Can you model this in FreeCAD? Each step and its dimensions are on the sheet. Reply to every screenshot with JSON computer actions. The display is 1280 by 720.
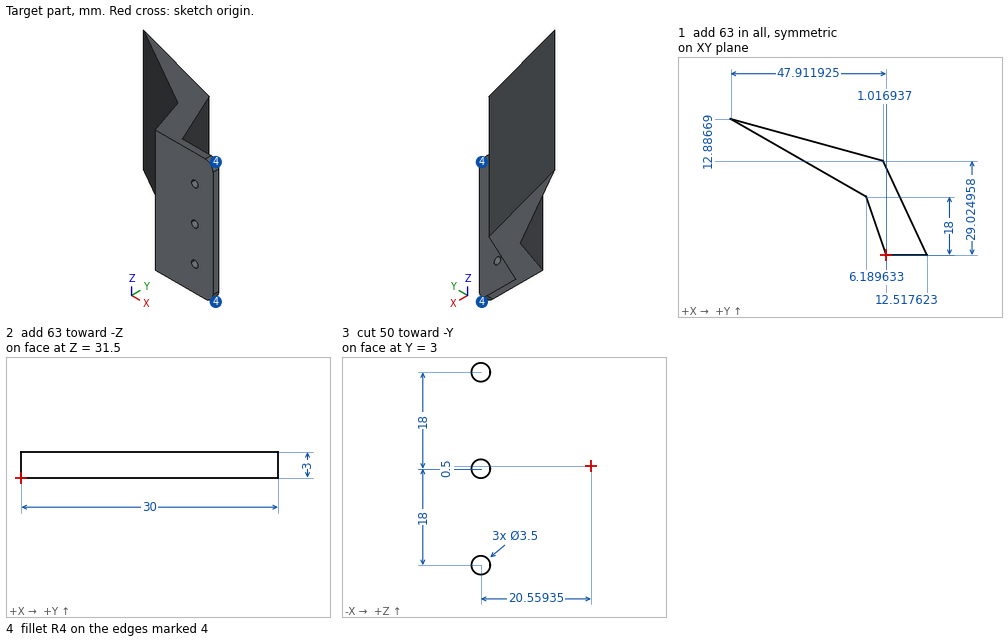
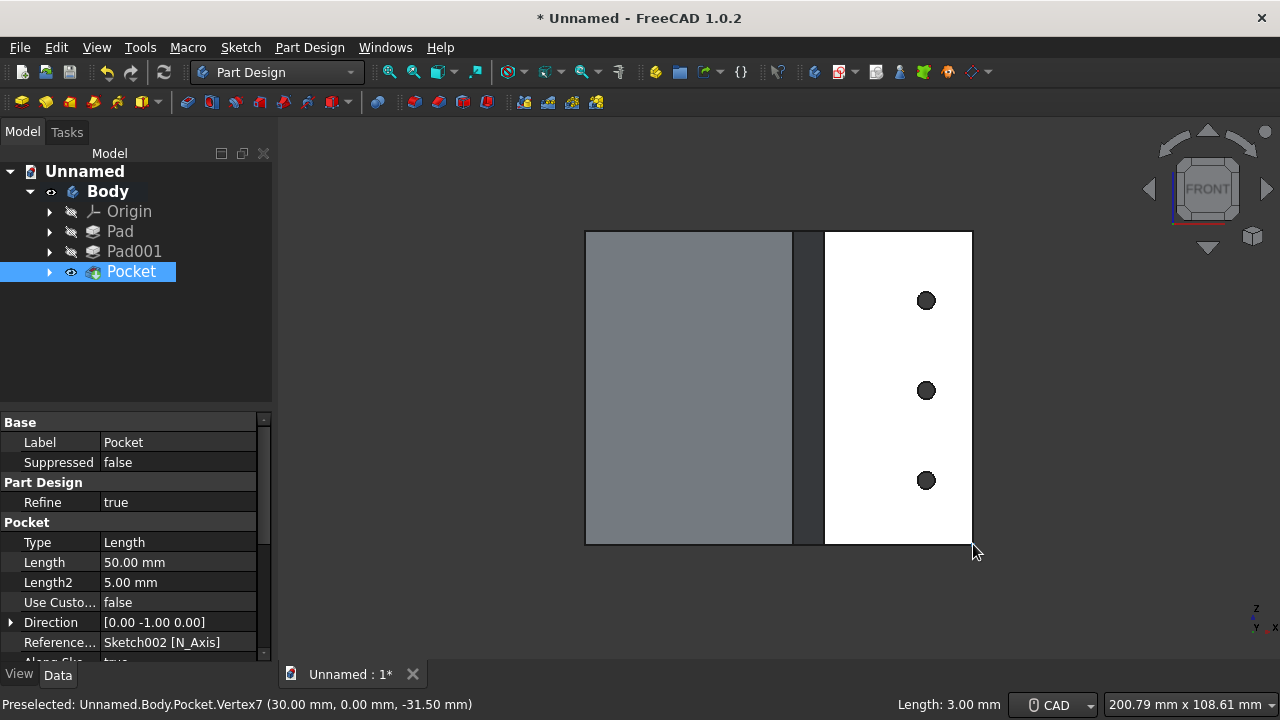
{"action": "key", "text": "3"}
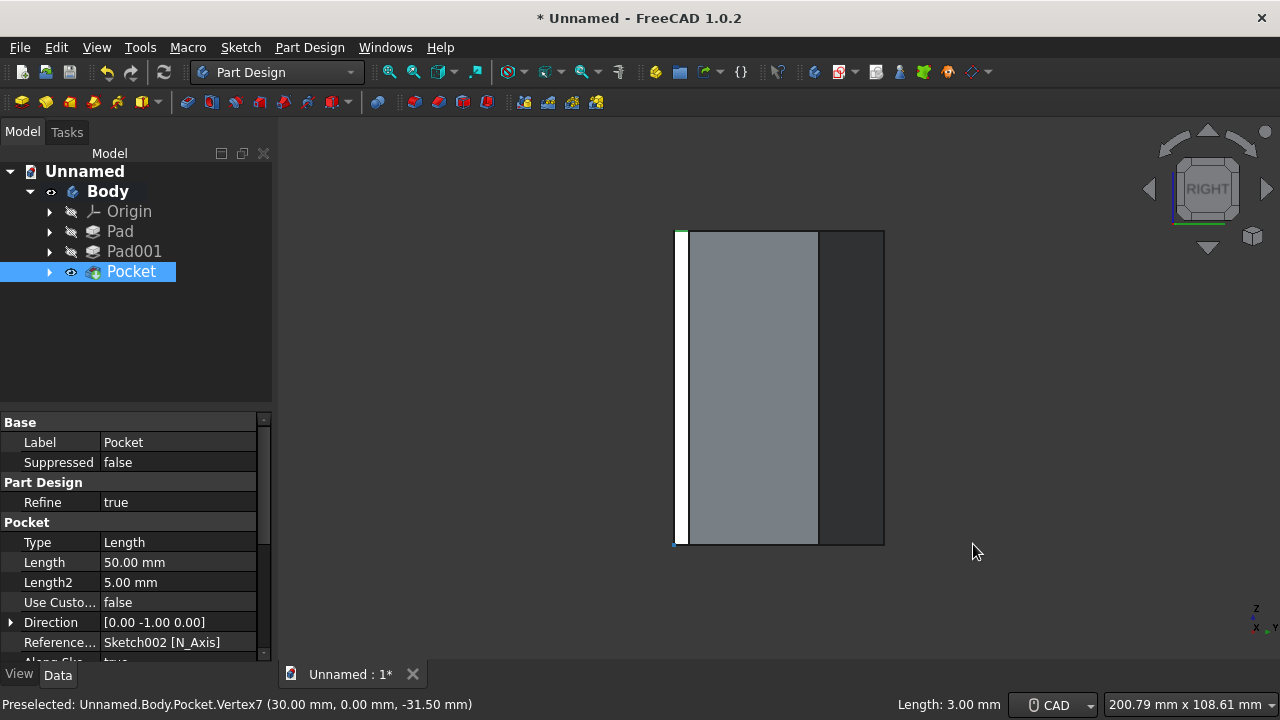
{"action": "left_click", "coordinate": [682, 544], "text": "ctrl"}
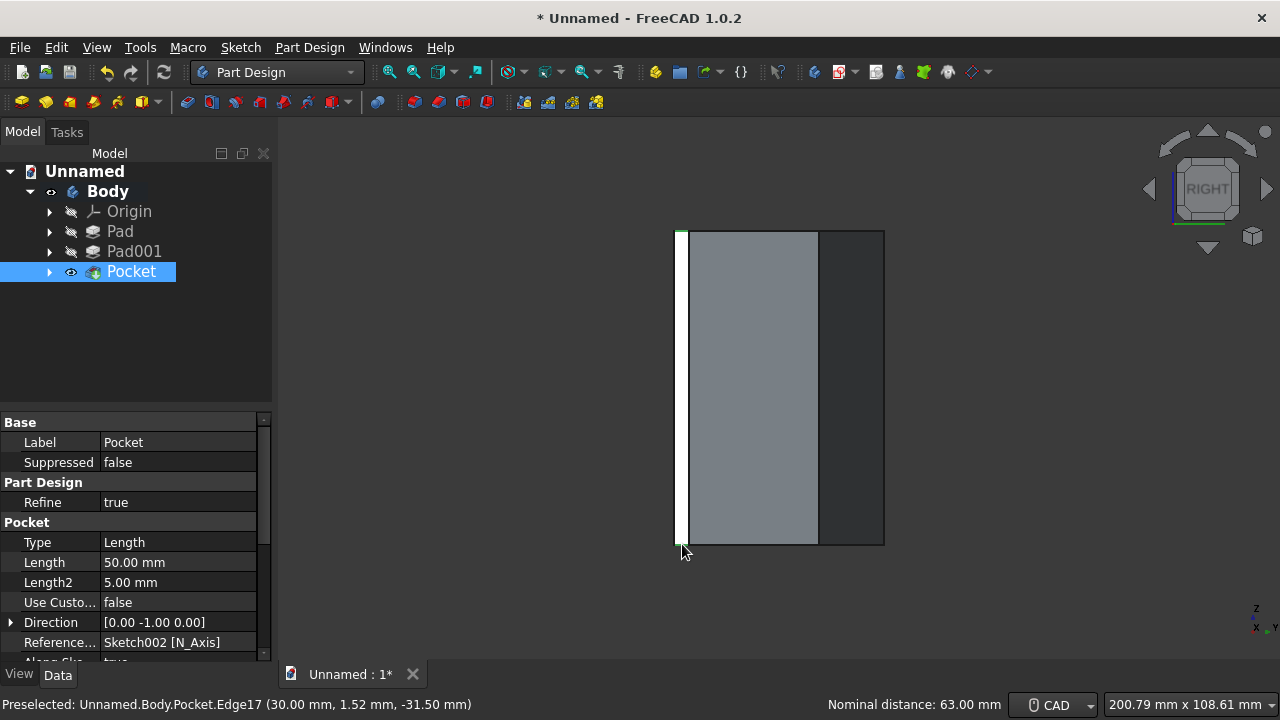
{"action": "left_click", "coordinate": [416, 102]}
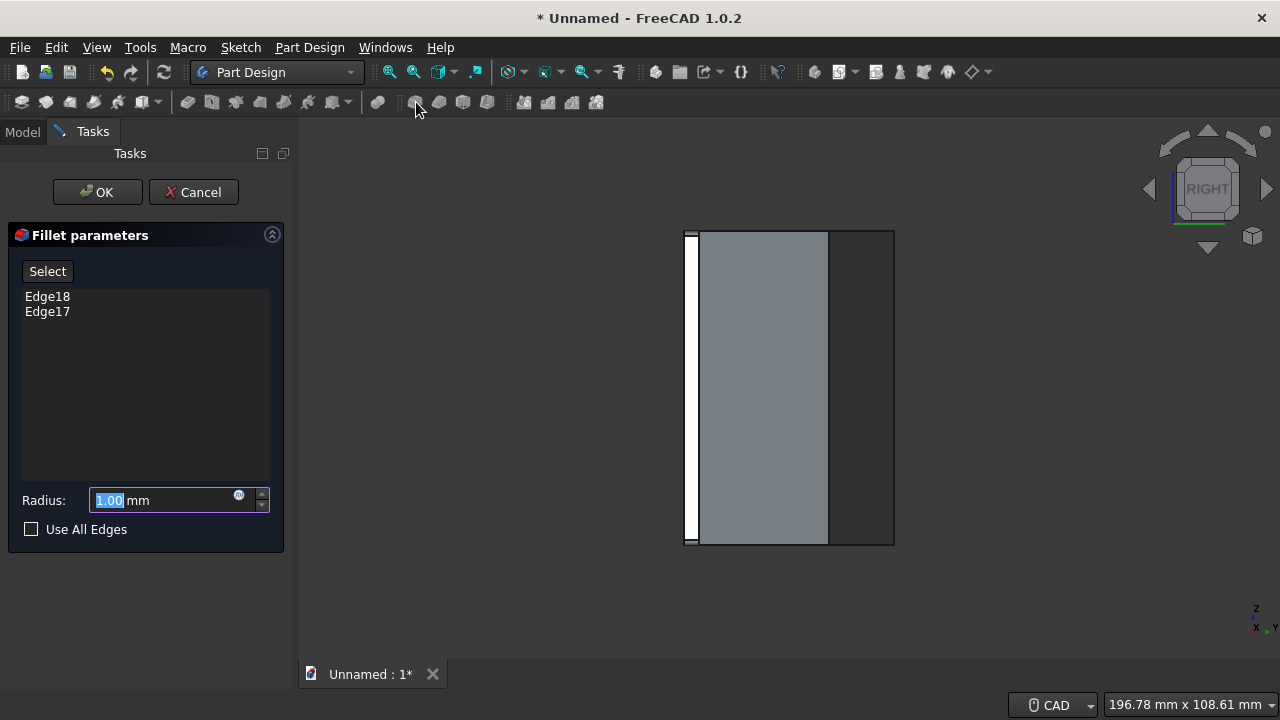
{"action": "type", "text": "4"}
{"action": "key", "text": "Tab"}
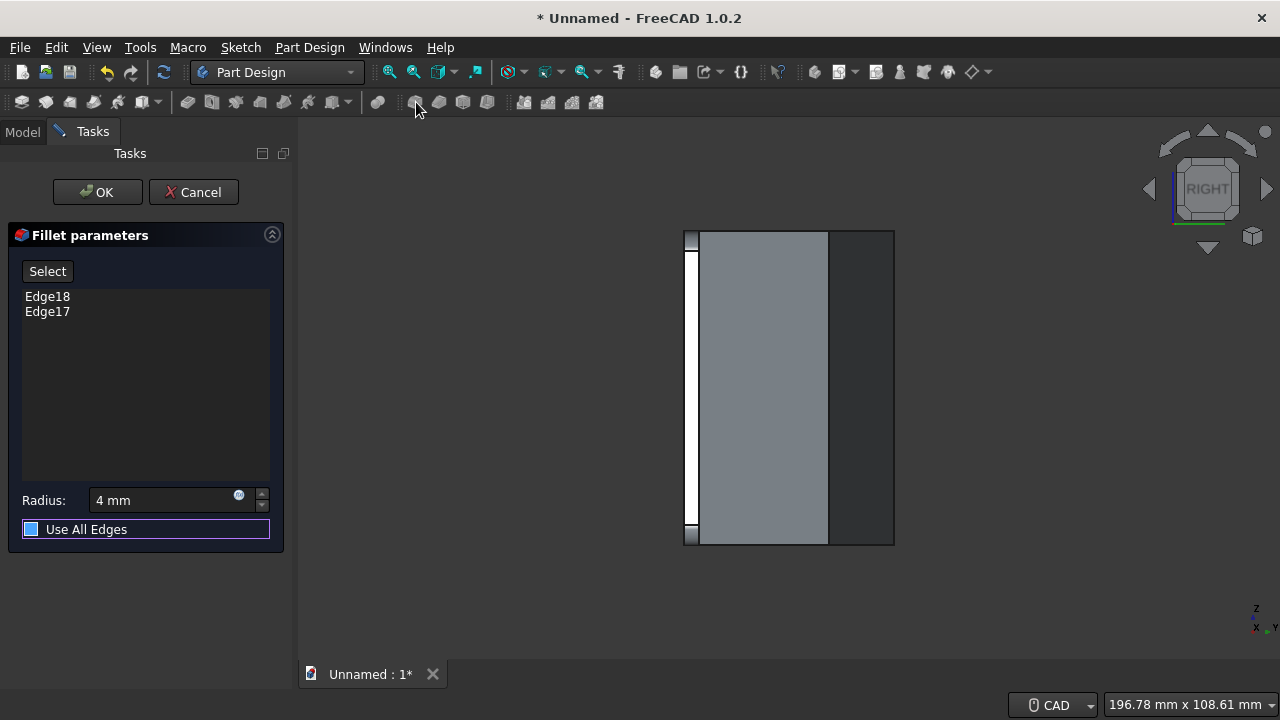
{"action": "left_click", "coordinate": [98, 192]}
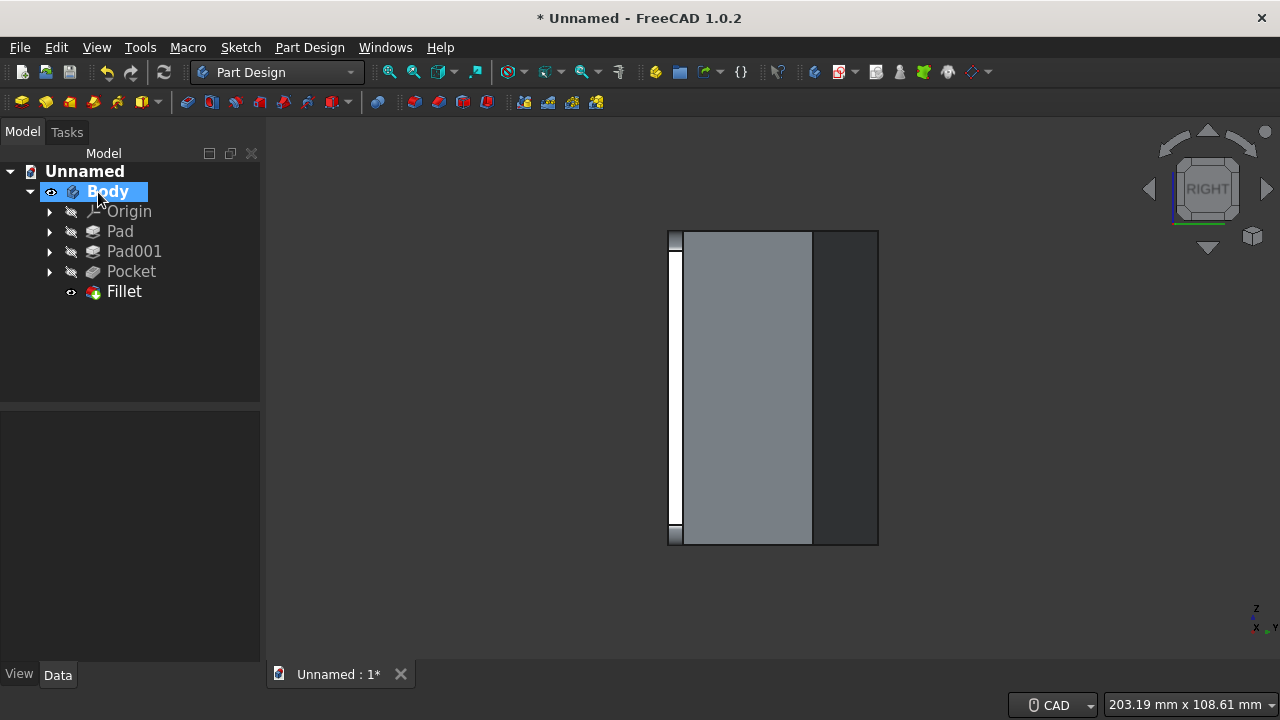
{"action": "key", "text": "0"}